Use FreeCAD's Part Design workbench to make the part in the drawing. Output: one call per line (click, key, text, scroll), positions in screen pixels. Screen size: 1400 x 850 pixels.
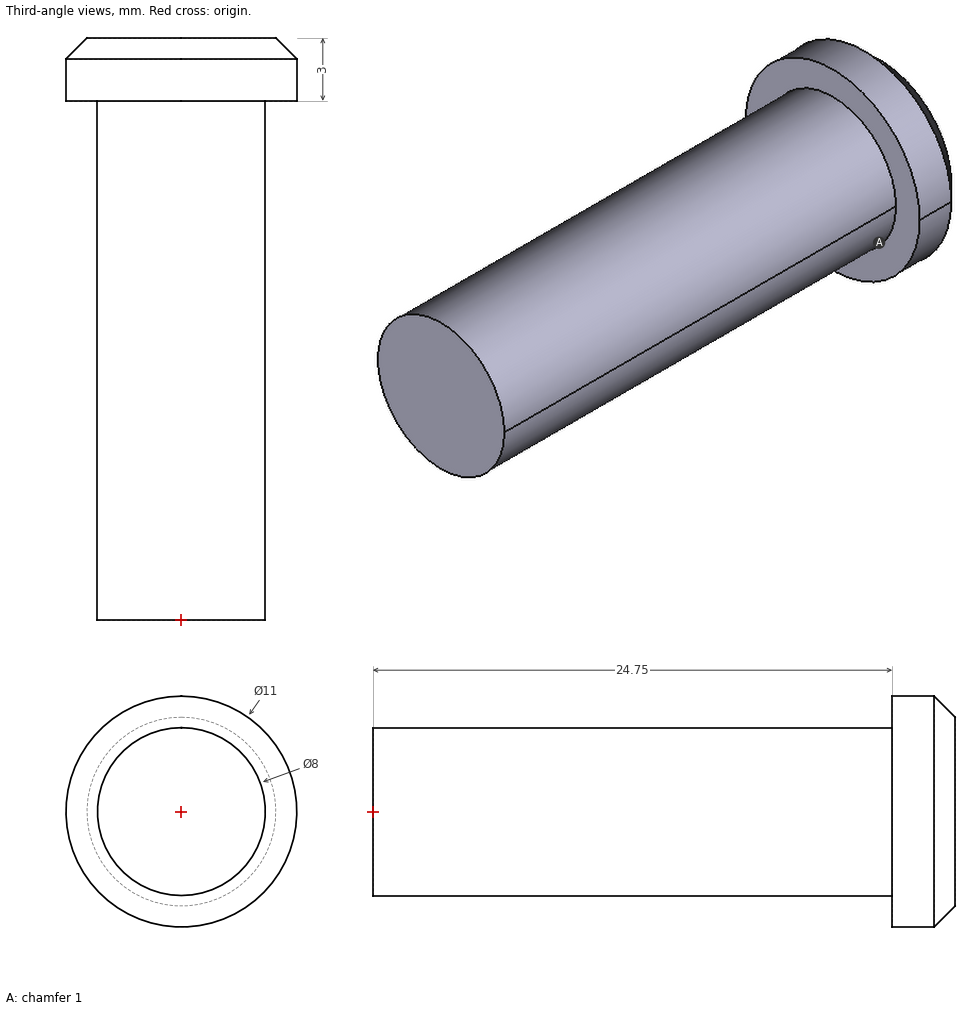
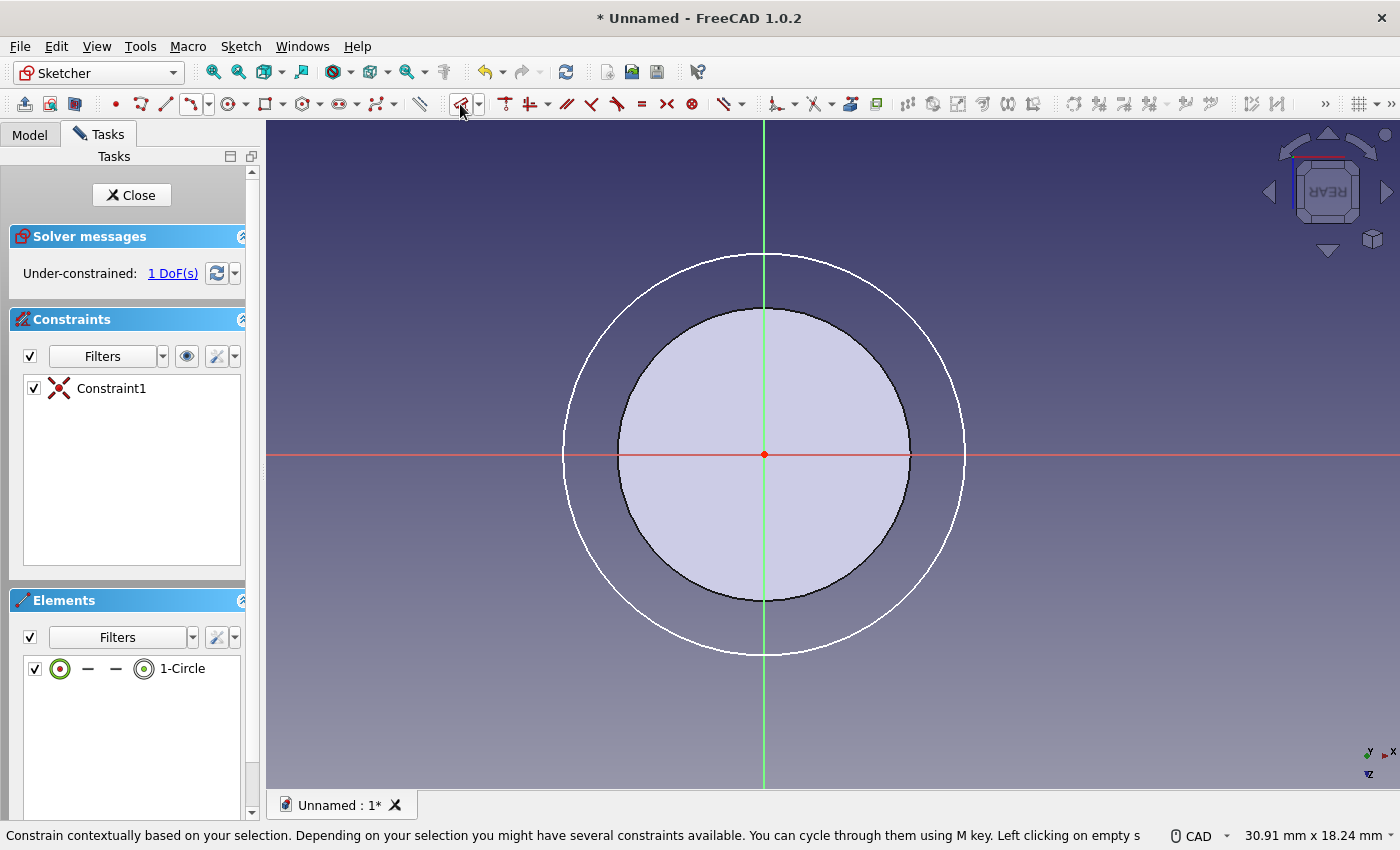
click(906, 312)
click(929, 289)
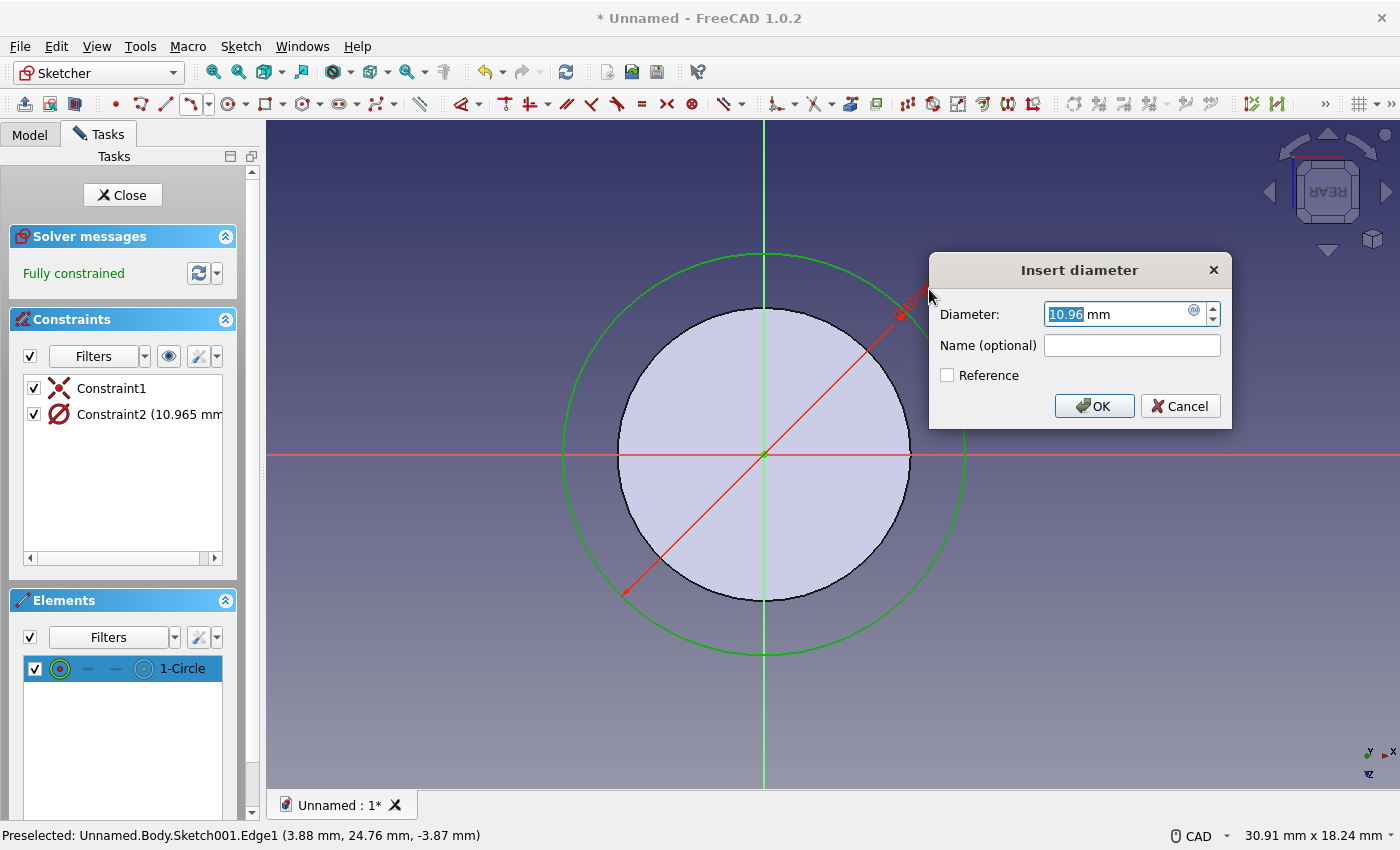
text(11)
key(Return)
key(Escape)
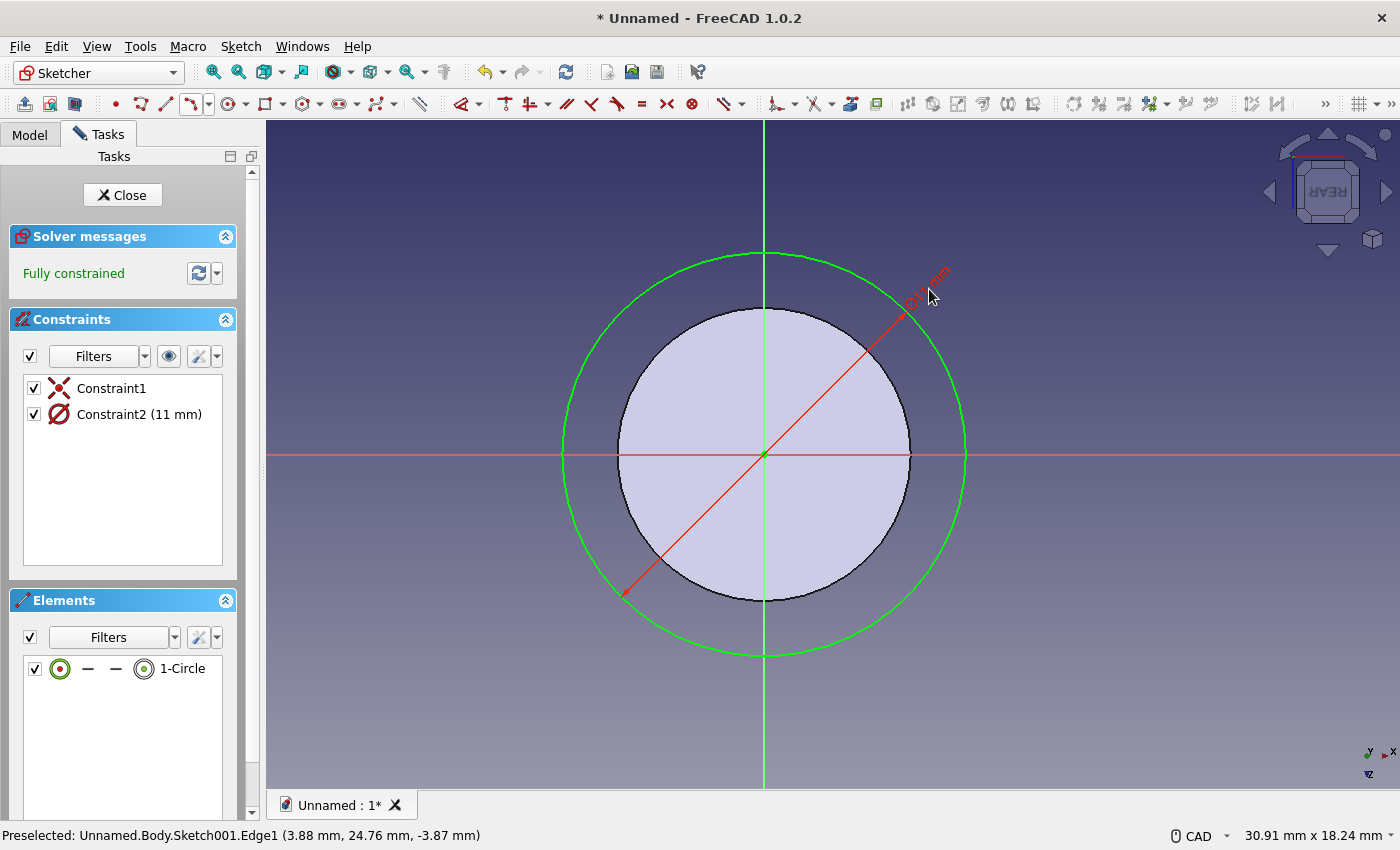
click(123, 195)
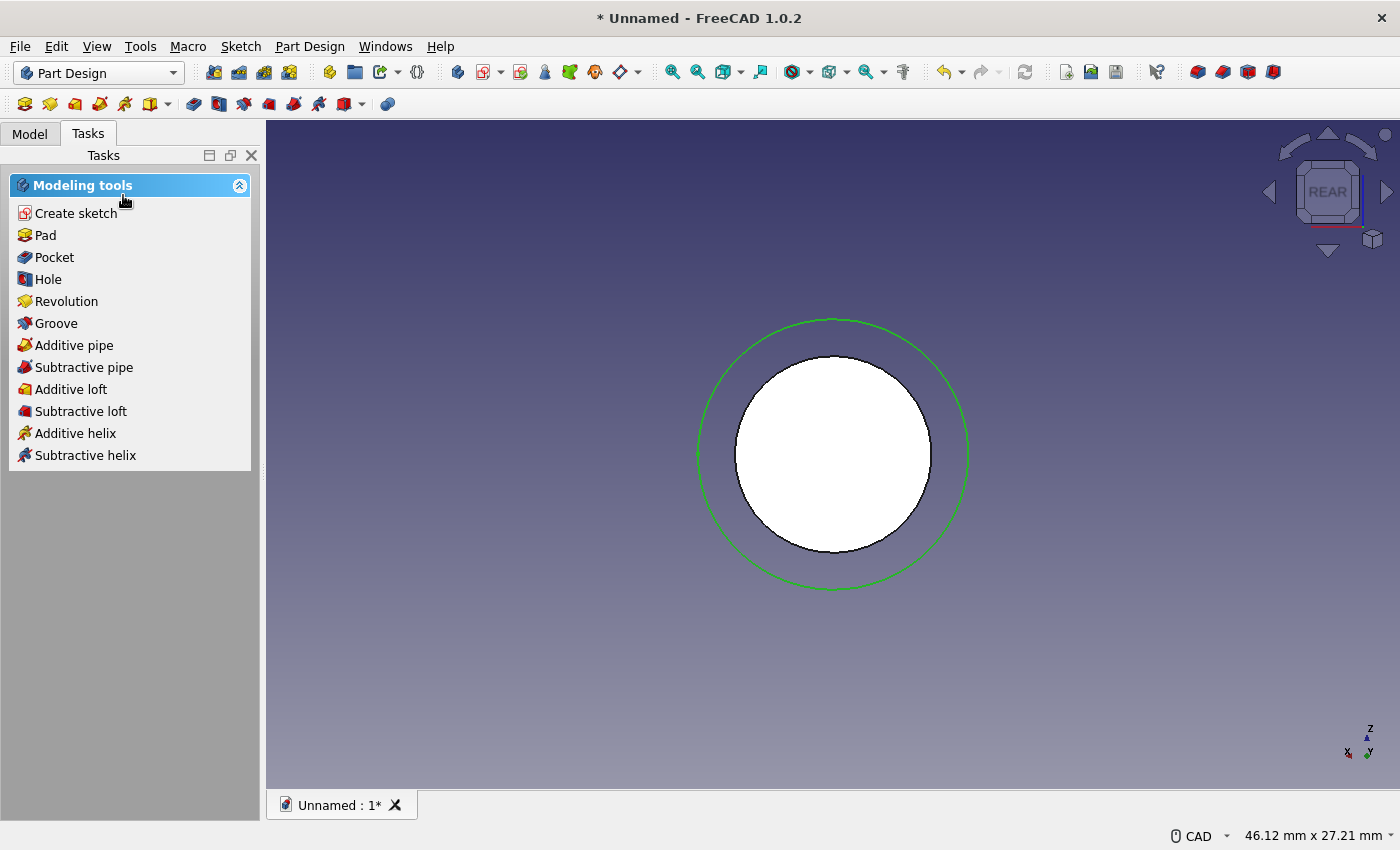
click(25, 104)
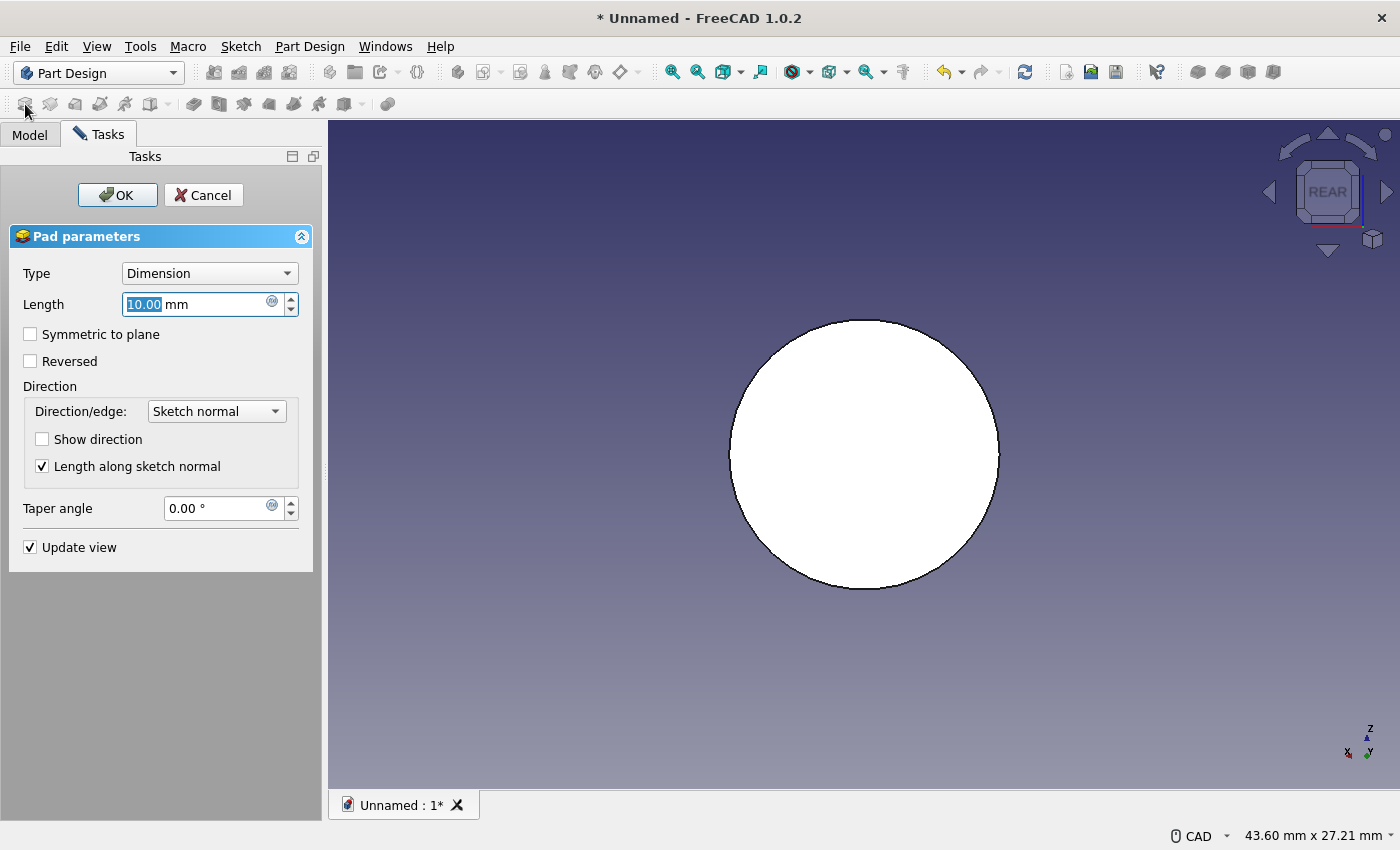
text(3)
key(Tab)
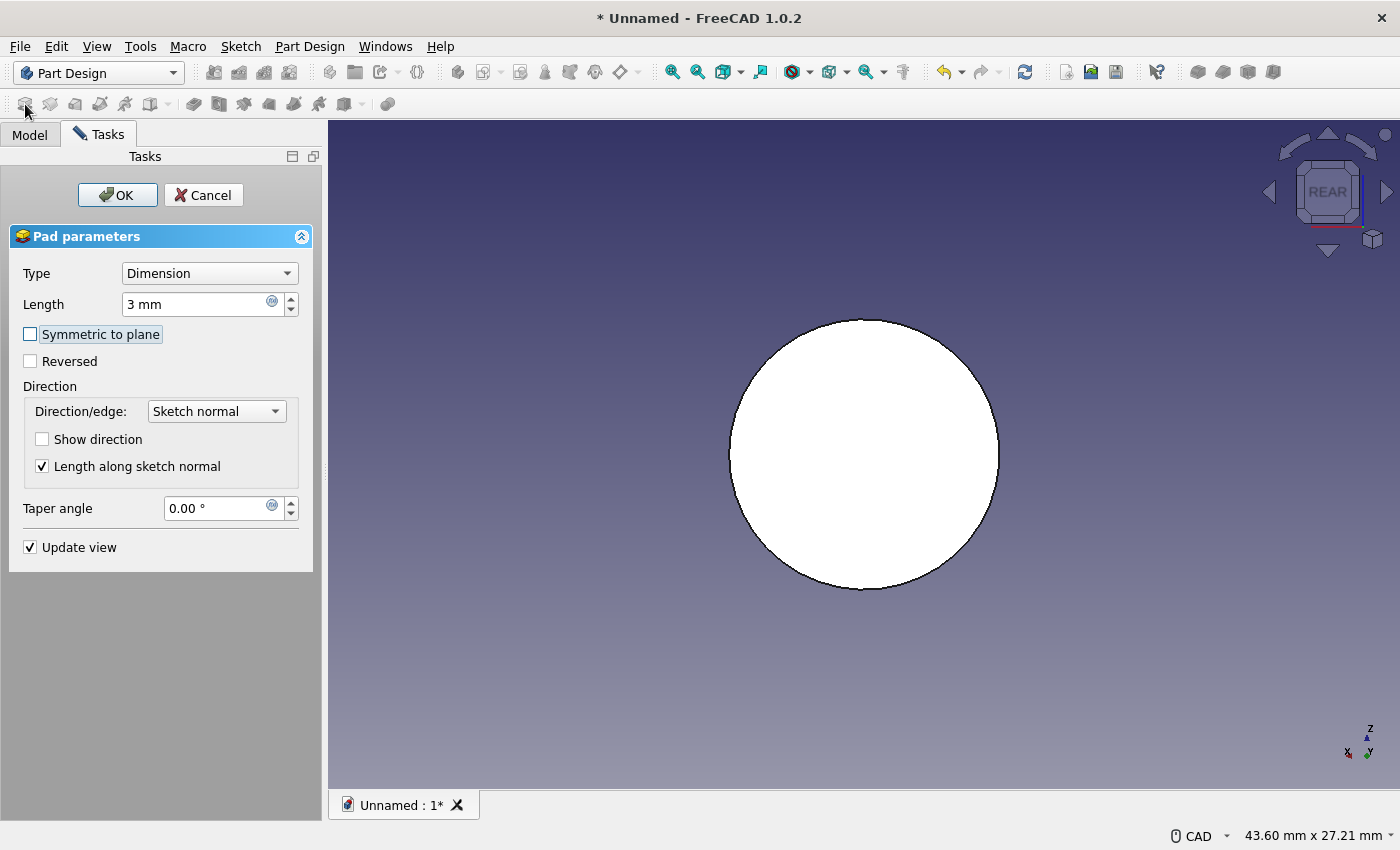
click(118, 195)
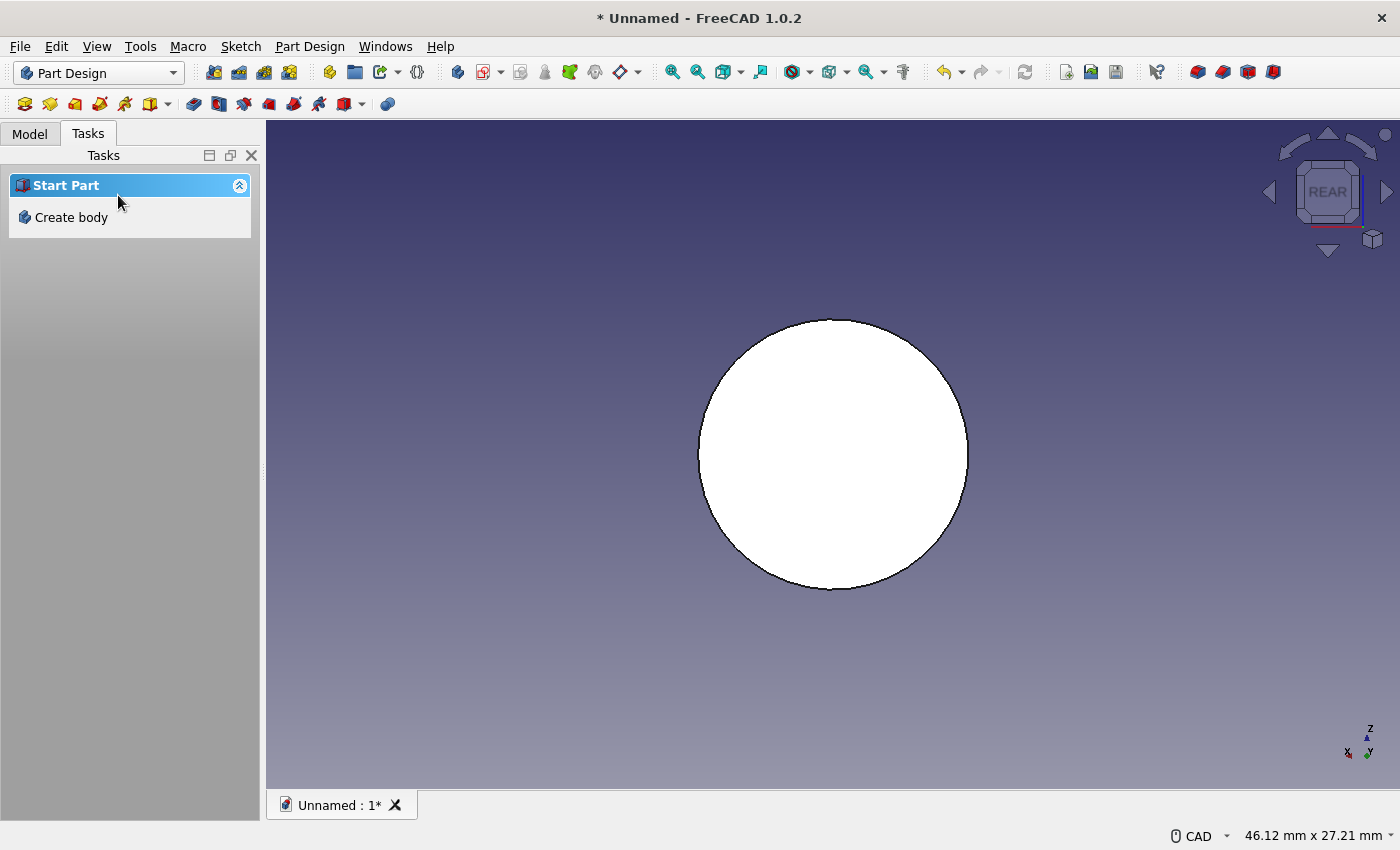
click(673, 72)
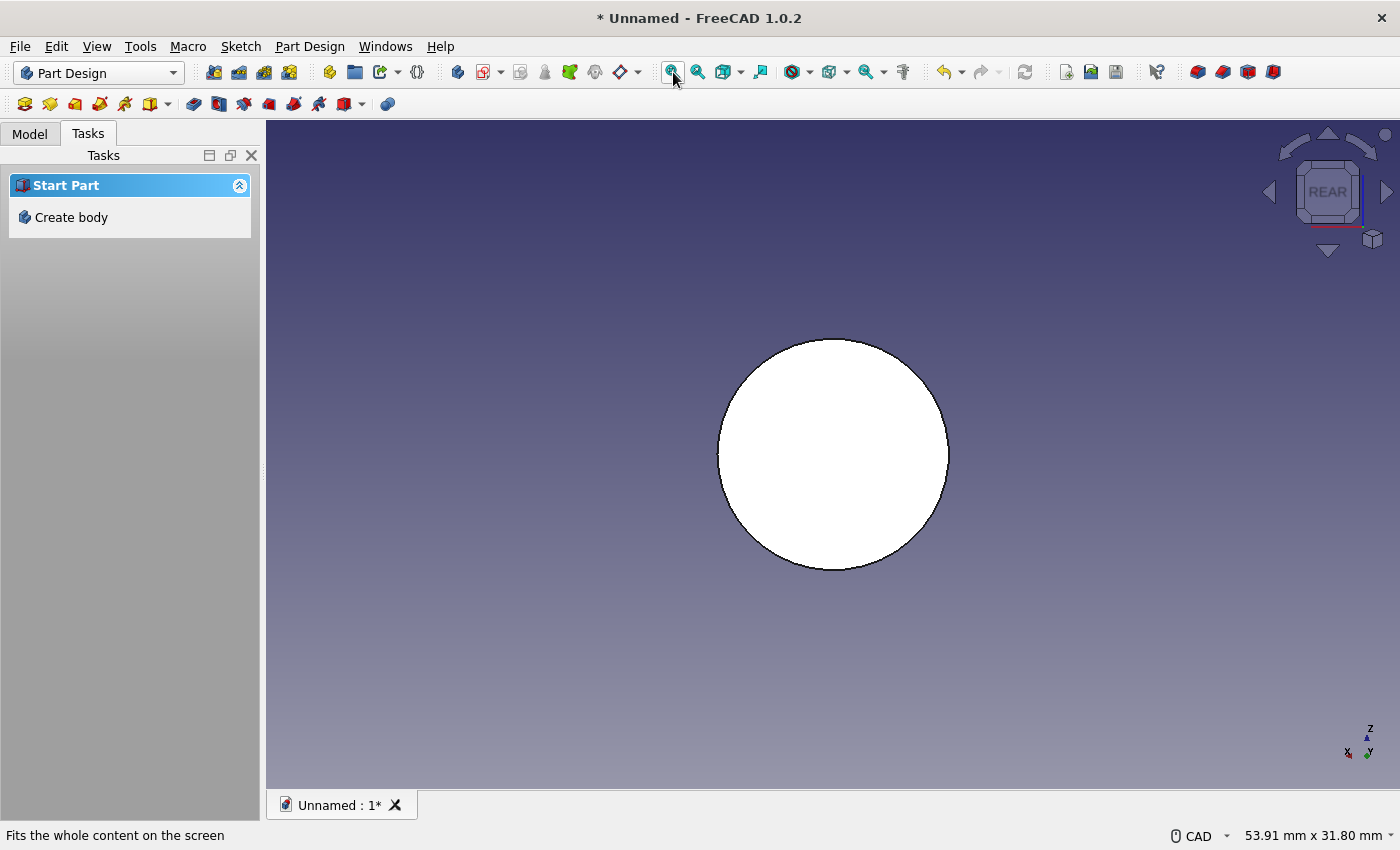
click(949, 453)